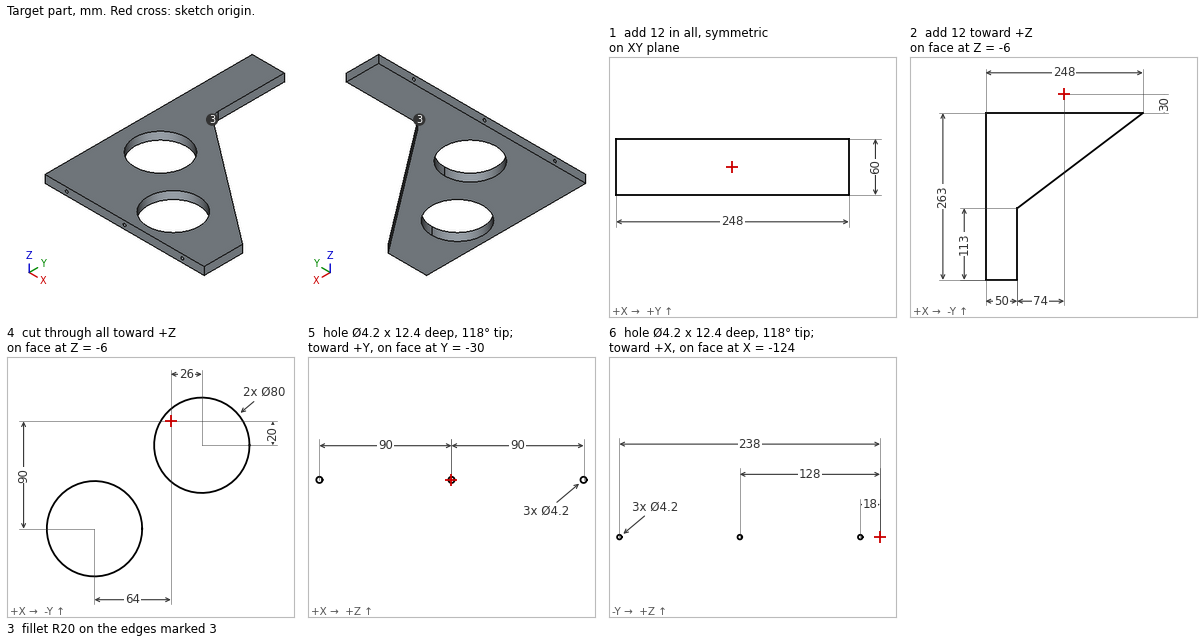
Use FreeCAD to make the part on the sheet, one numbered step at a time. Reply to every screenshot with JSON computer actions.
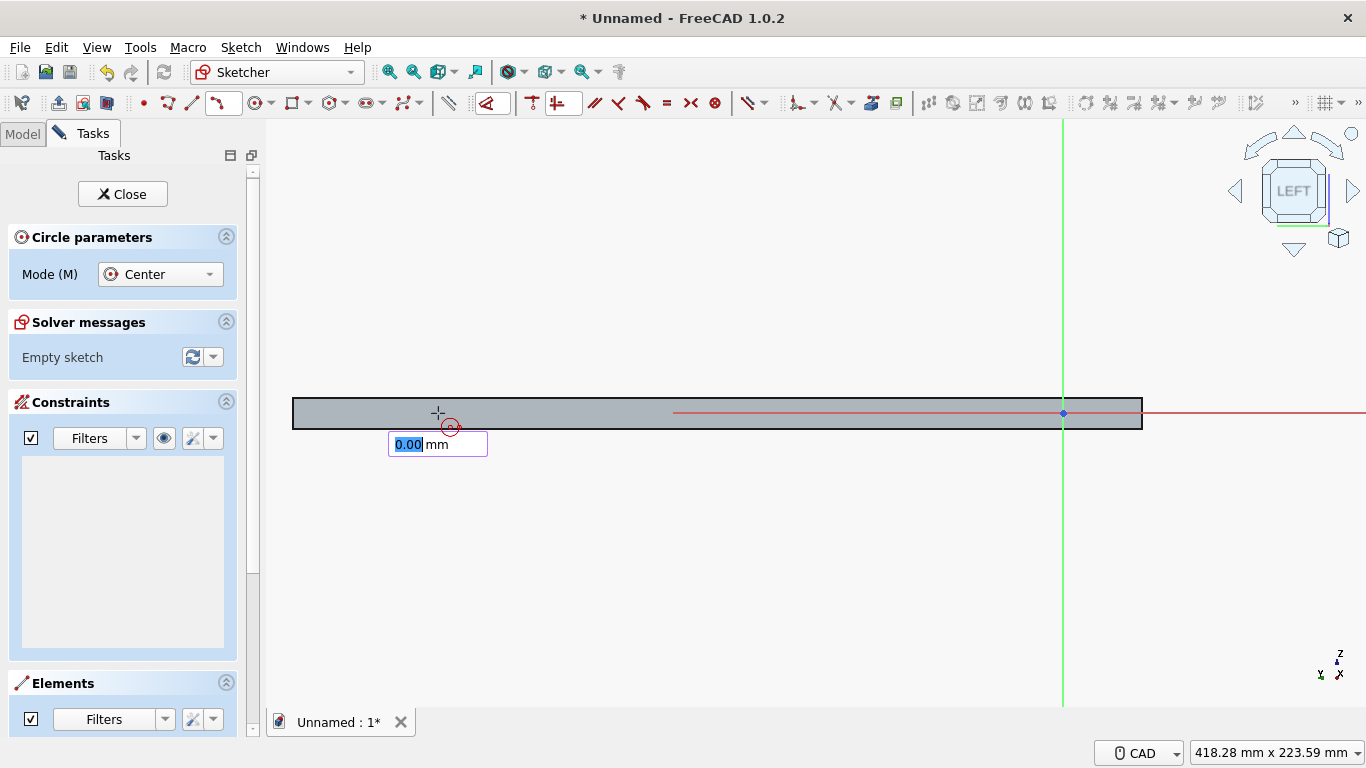
{"action": "scroll", "coordinate": [439, 408], "scroll_direction": "up", "scroll_amount": 6}
{"action": "mouse_move", "coordinate": [440, 408]}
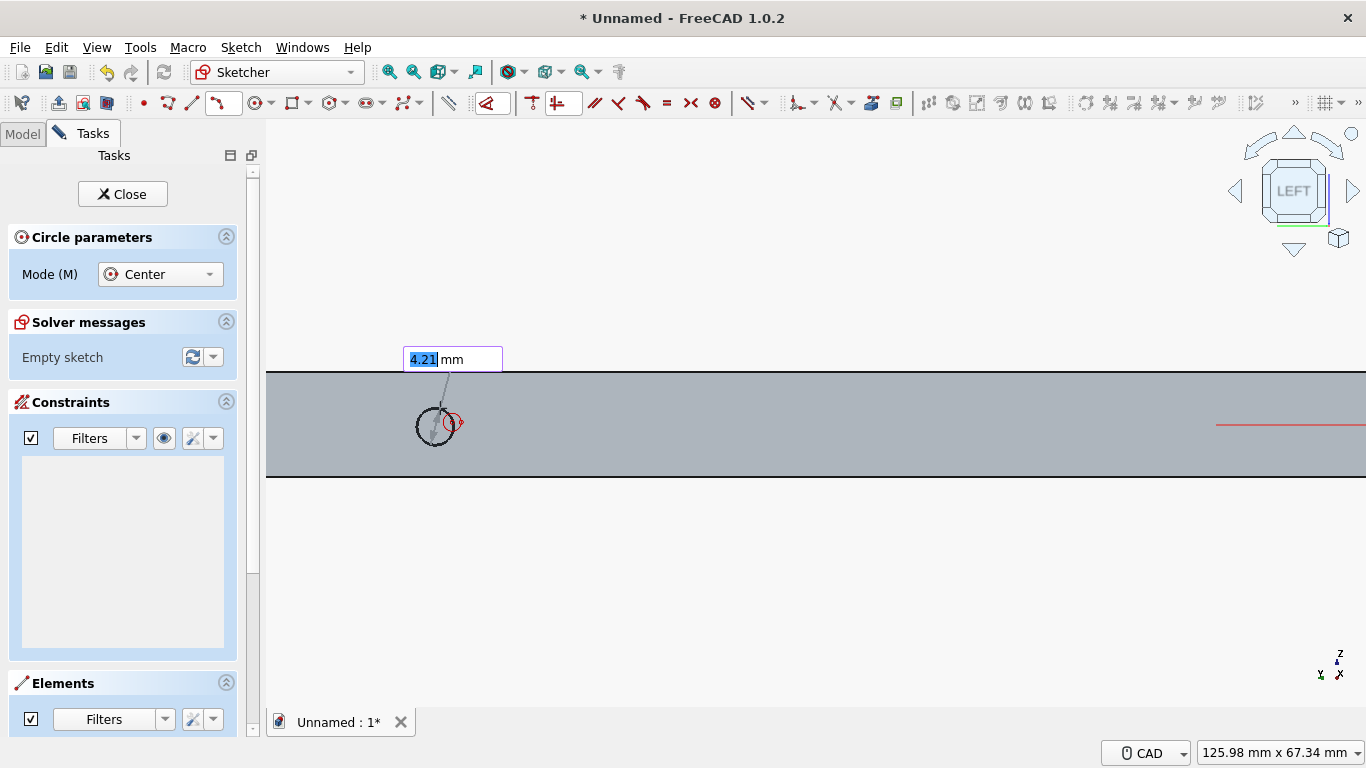
{"action": "type", "text": "4.2"}
{"action": "key", "text": "Return"}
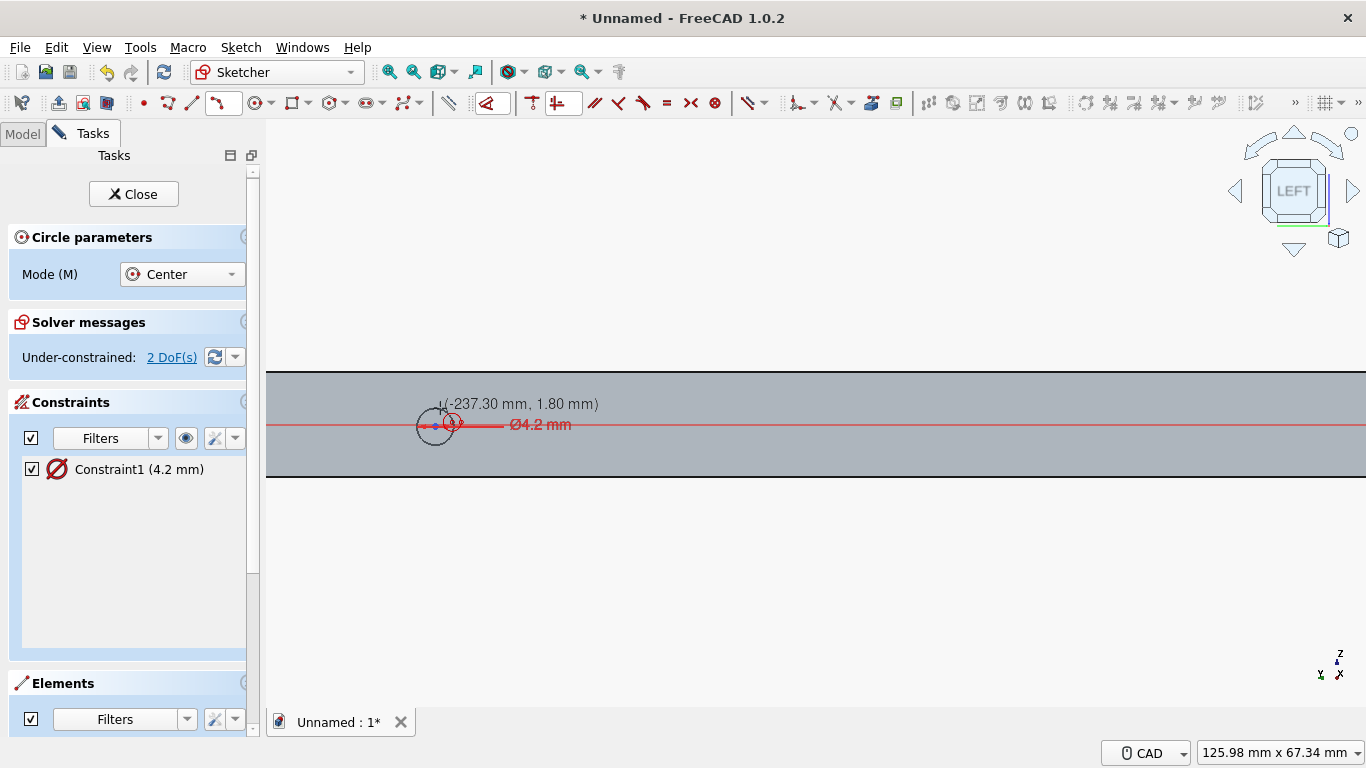
{"action": "scroll", "coordinate": [439, 408], "scroll_direction": "down", "scroll_amount": 6}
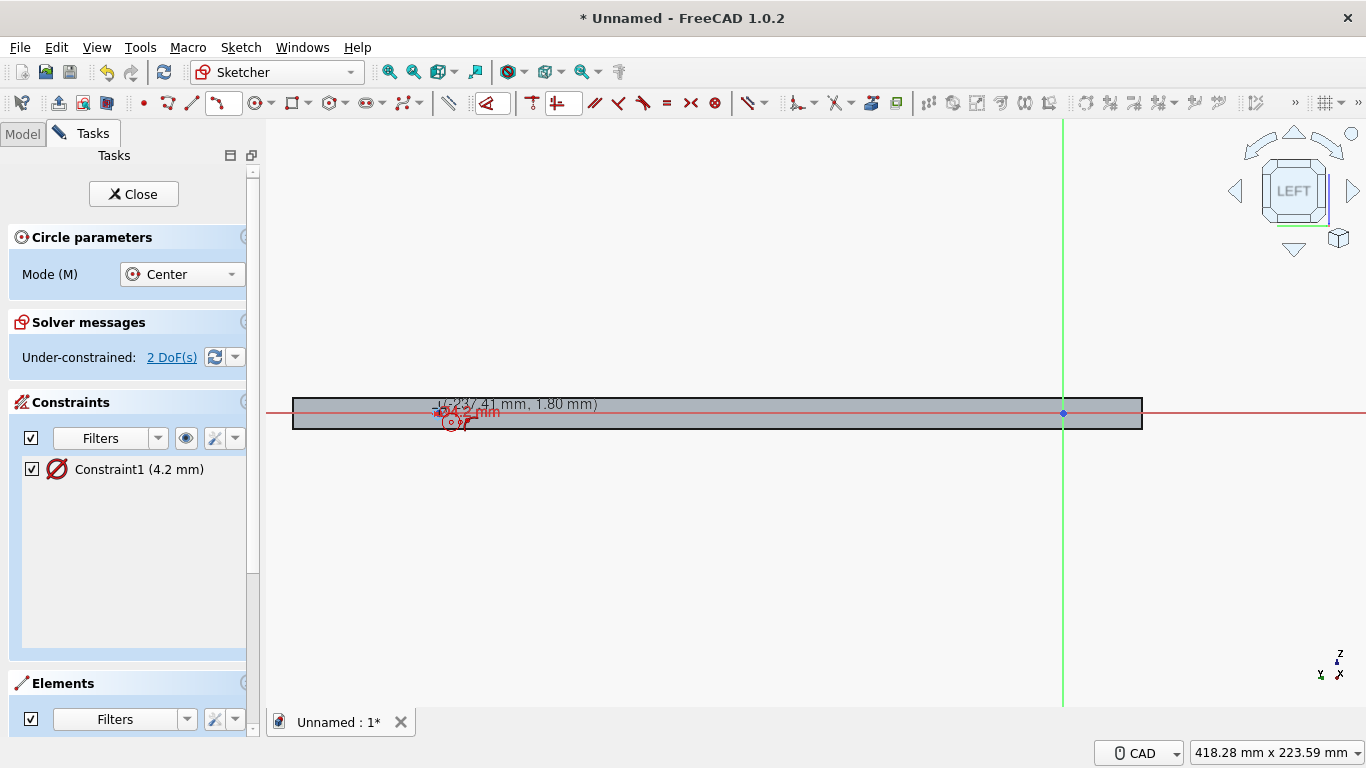
{"action": "scroll", "coordinate": [727, 413], "scroll_direction": "up", "scroll_amount": 8}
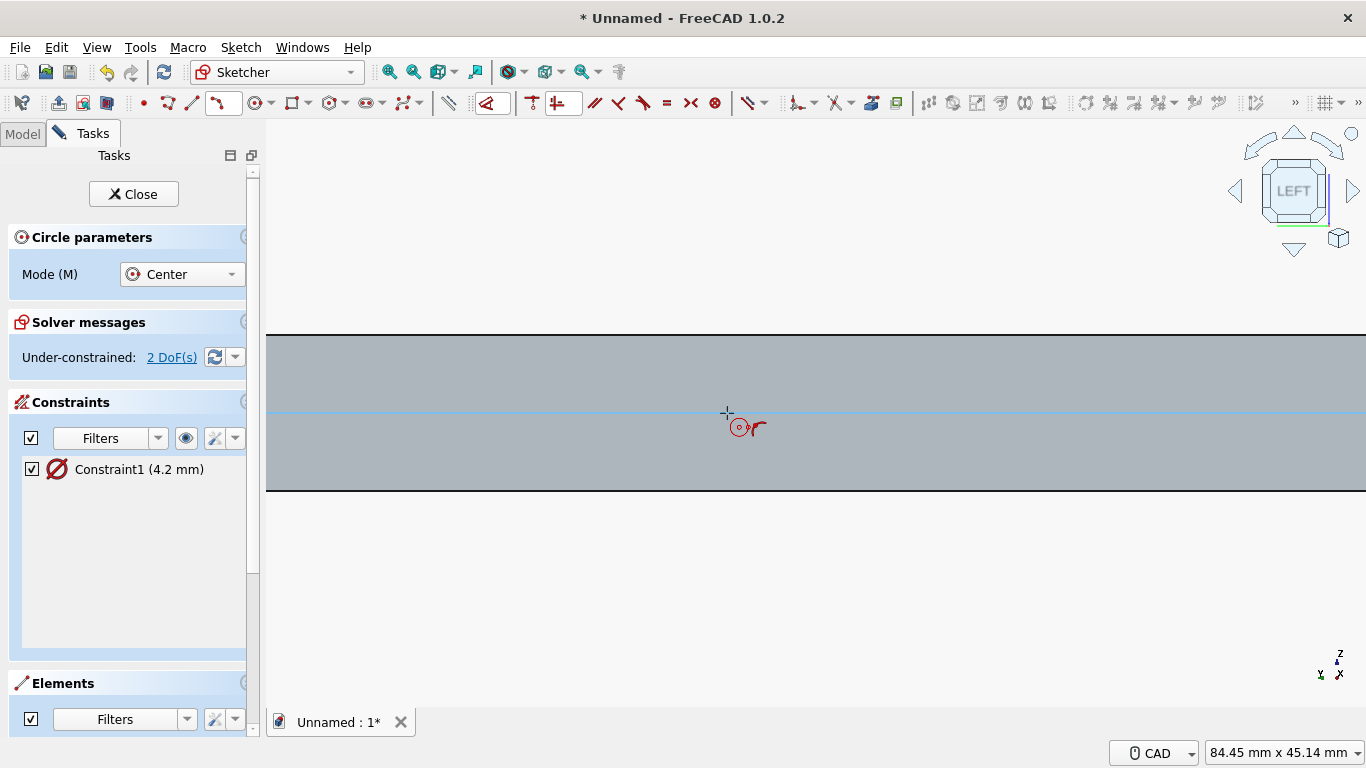
{"action": "scroll", "coordinate": [727, 413], "scroll_direction": "down", "scroll_amount": 8}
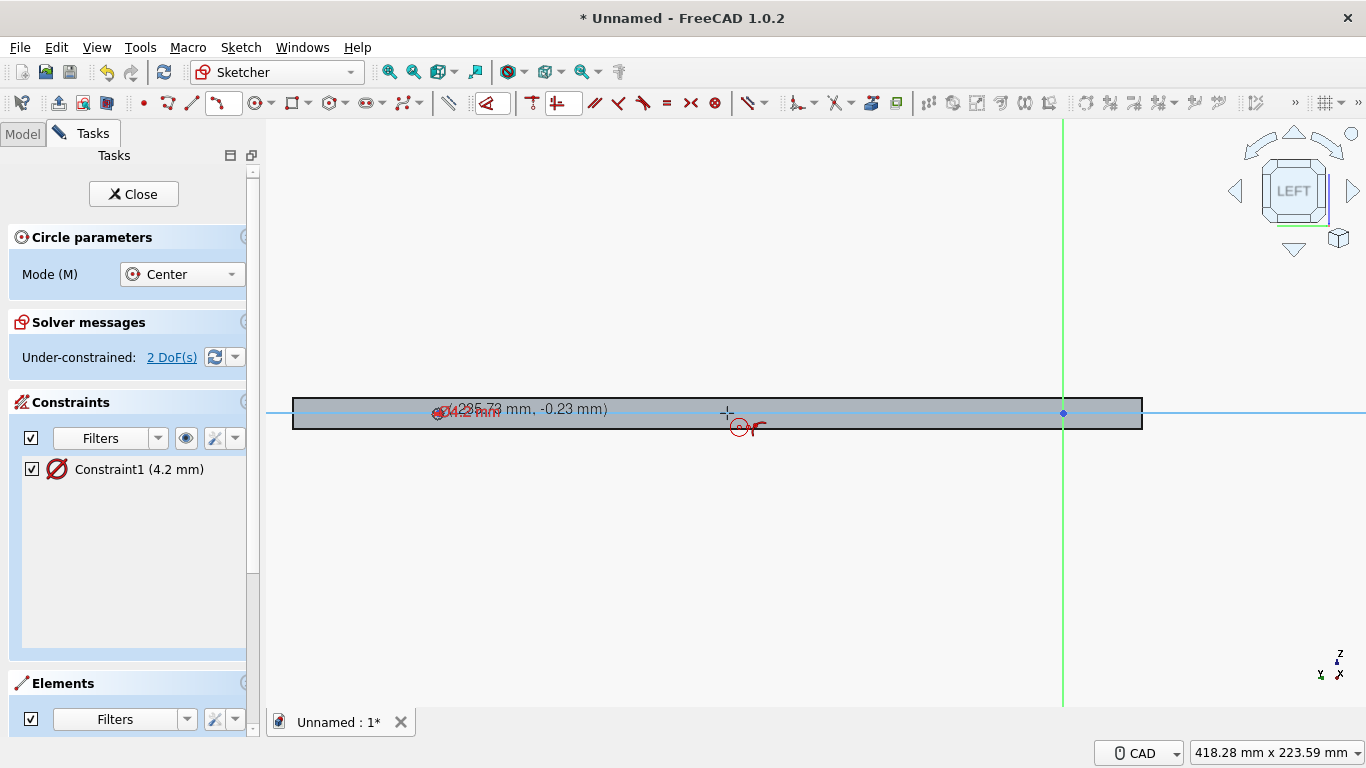
{"action": "left_click", "coordinate": [727, 413]}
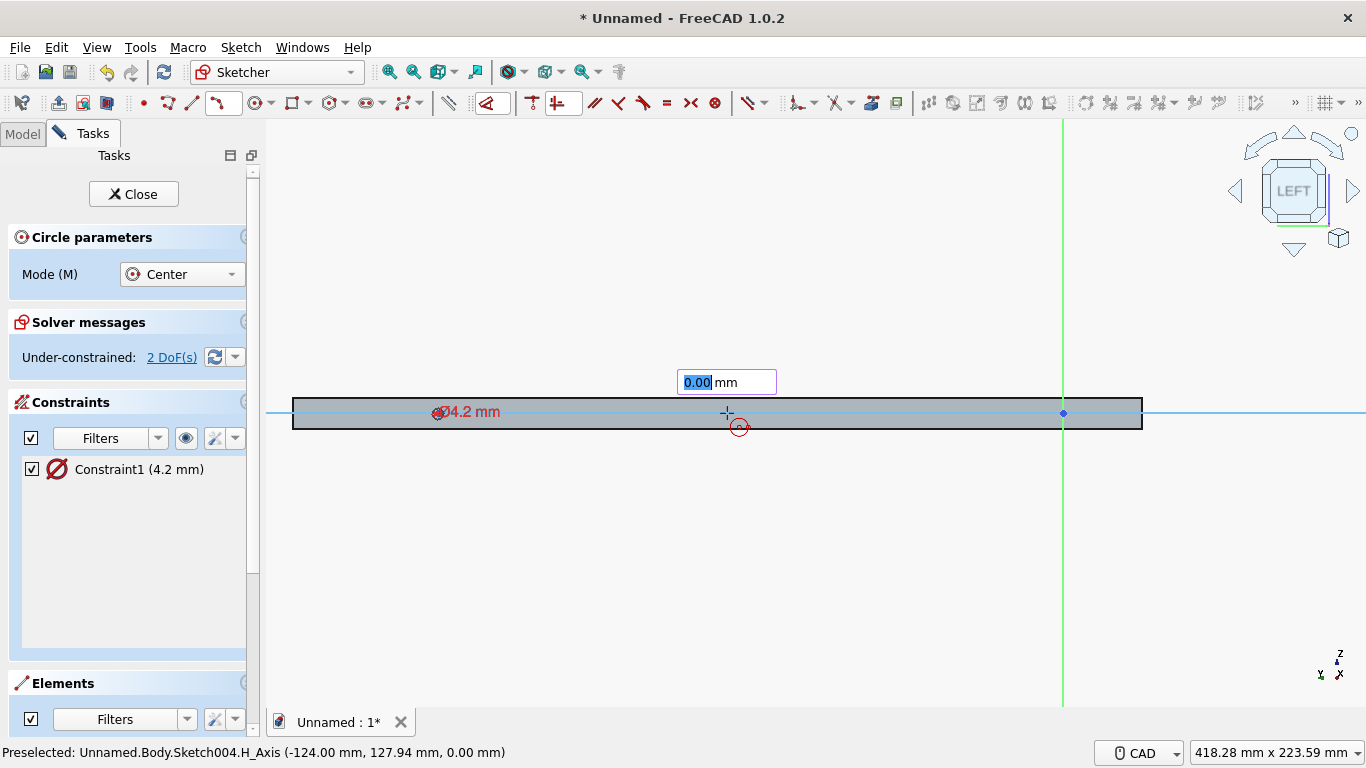
{"action": "scroll", "coordinate": [725, 419], "scroll_direction": "up", "scroll_amount": 6}
{"action": "mouse_move", "coordinate": [724, 416]}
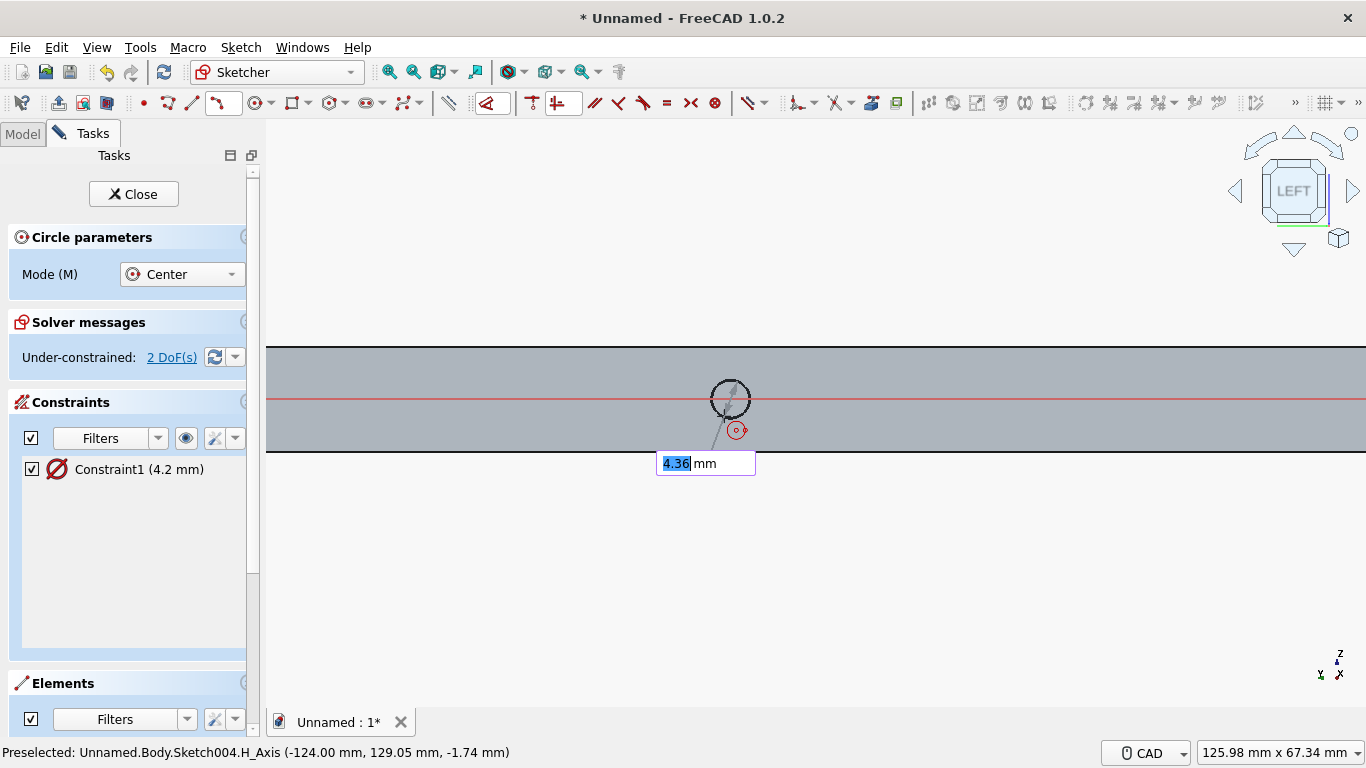
{"action": "type", "text": "4.2"}
{"action": "key", "text": "Return"}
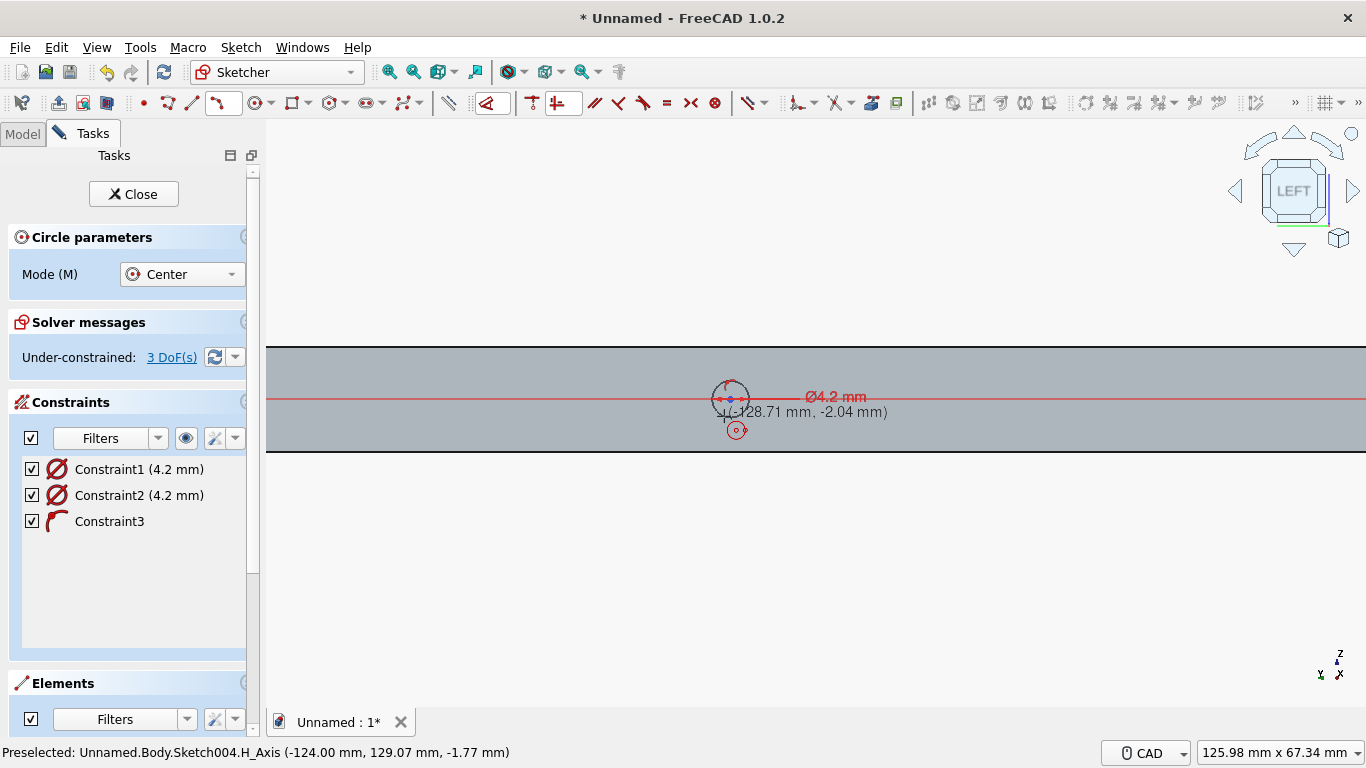
{"action": "scroll", "coordinate": [725, 419], "scroll_direction": "down", "scroll_amount": 6}